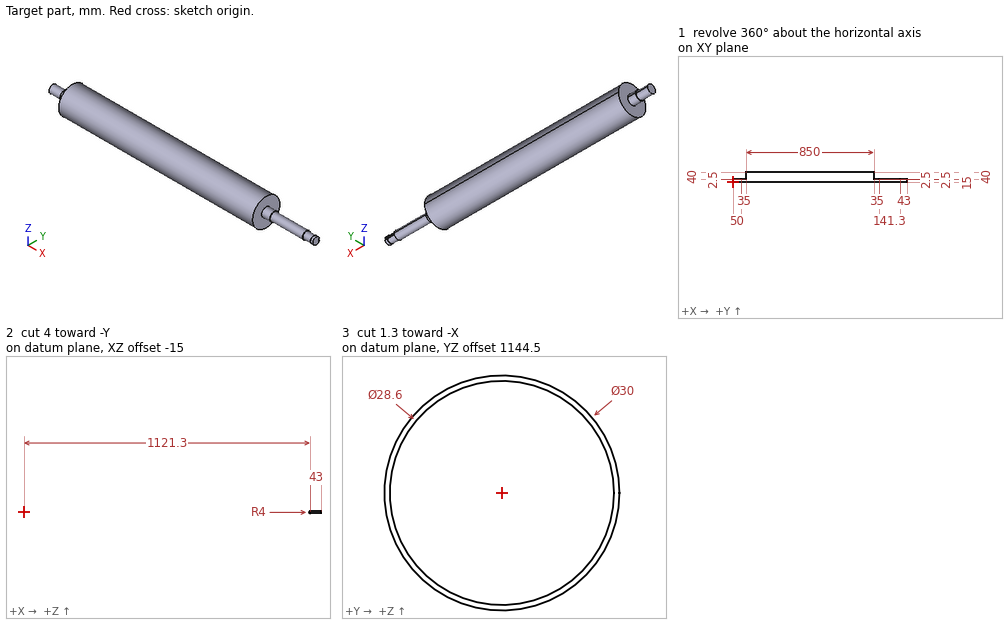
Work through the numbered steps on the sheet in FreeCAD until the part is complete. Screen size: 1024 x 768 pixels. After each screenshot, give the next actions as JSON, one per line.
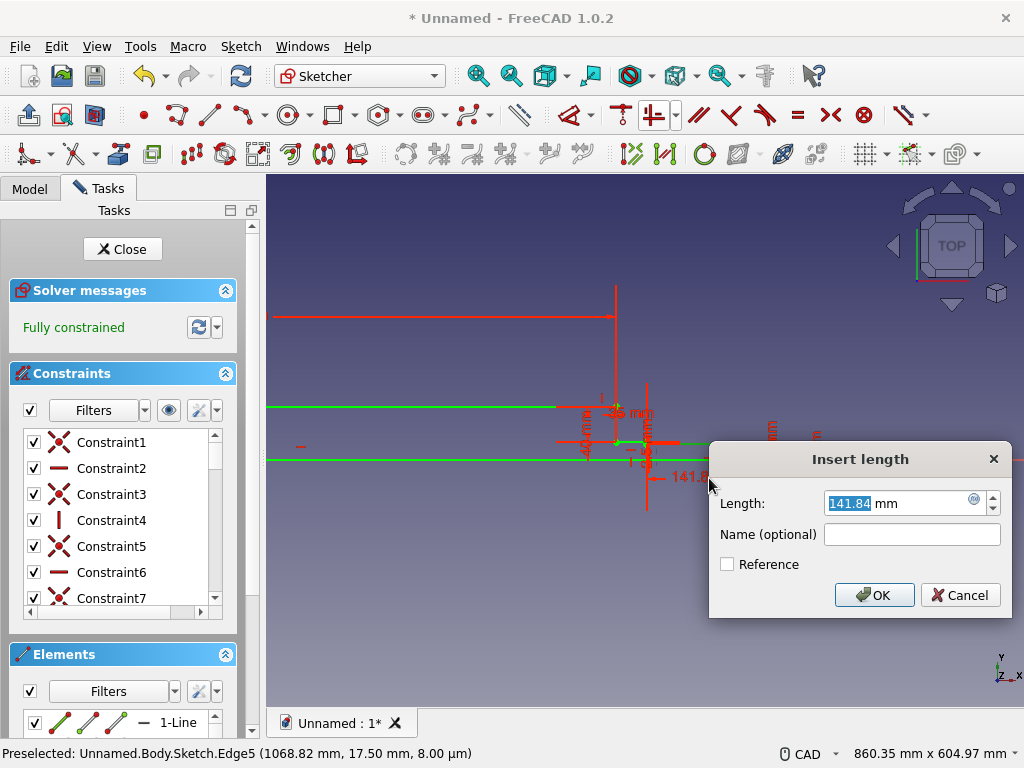
{"action": "type", "text": "141.3"}
{"action": "key", "text": "Return"}
{"action": "key", "text": "Escape"}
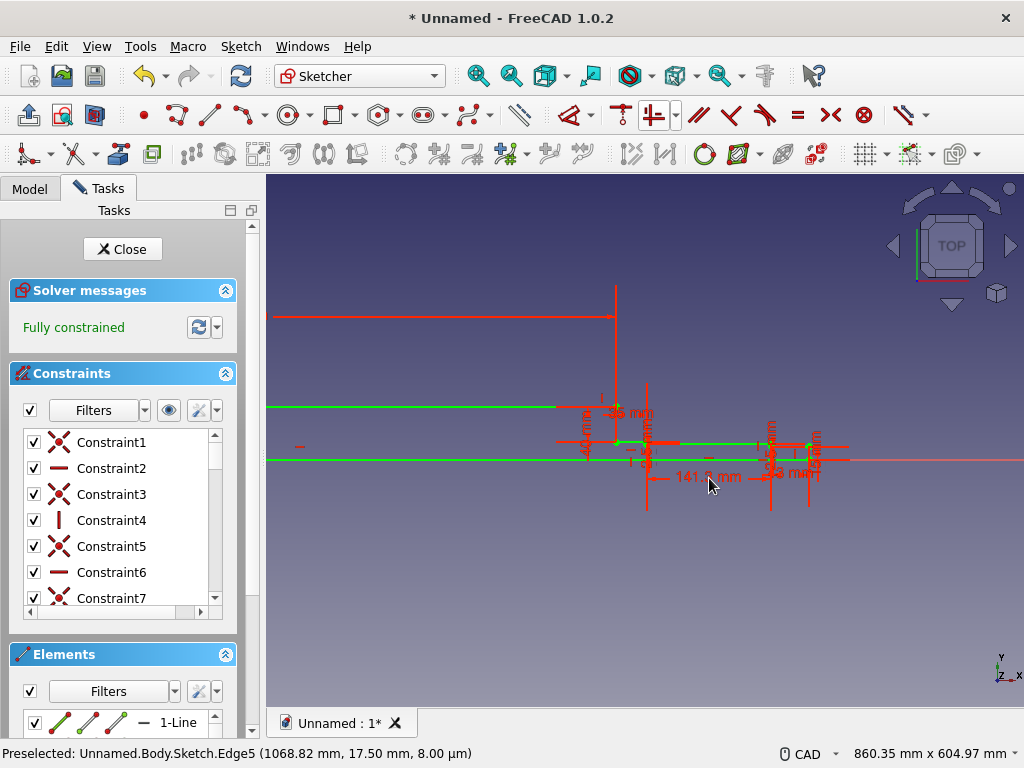
{"action": "left_click", "coordinate": [123, 249]}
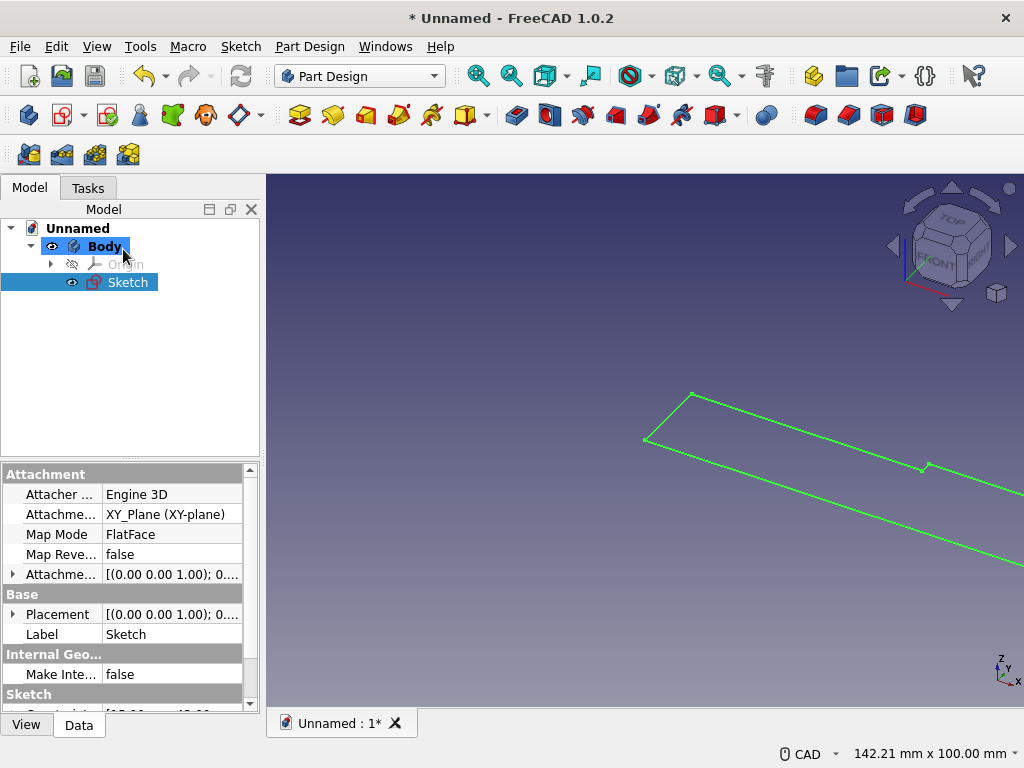
{"action": "left_click", "coordinate": [333, 116]}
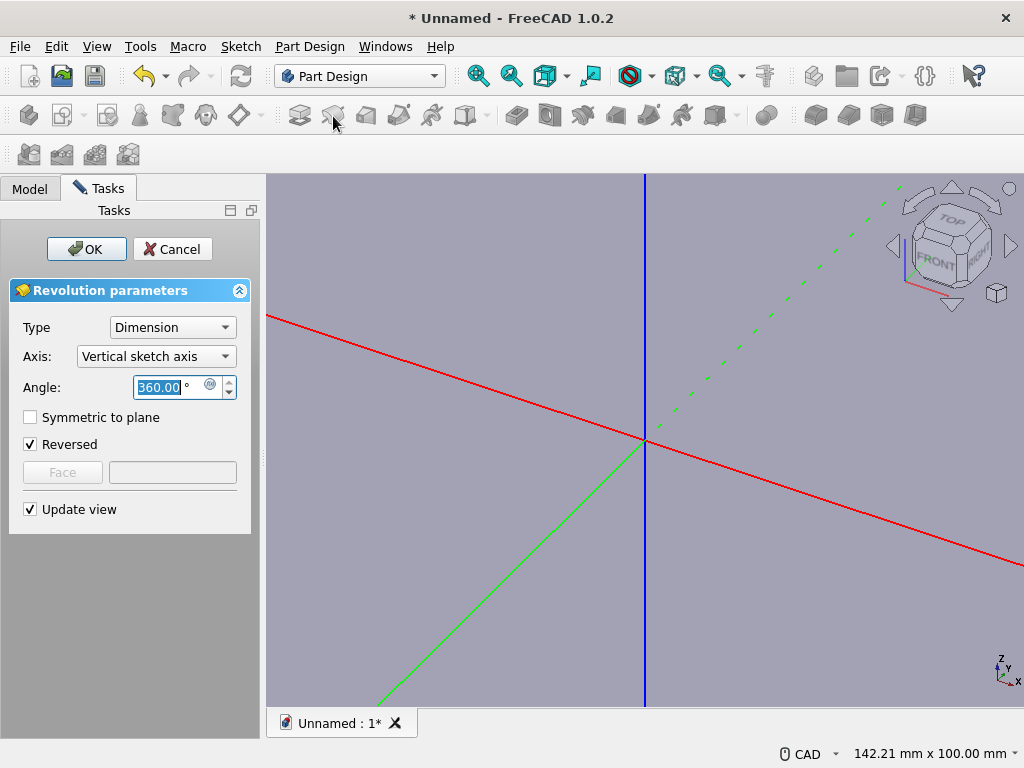
{"action": "left_click", "coordinate": [157, 356]}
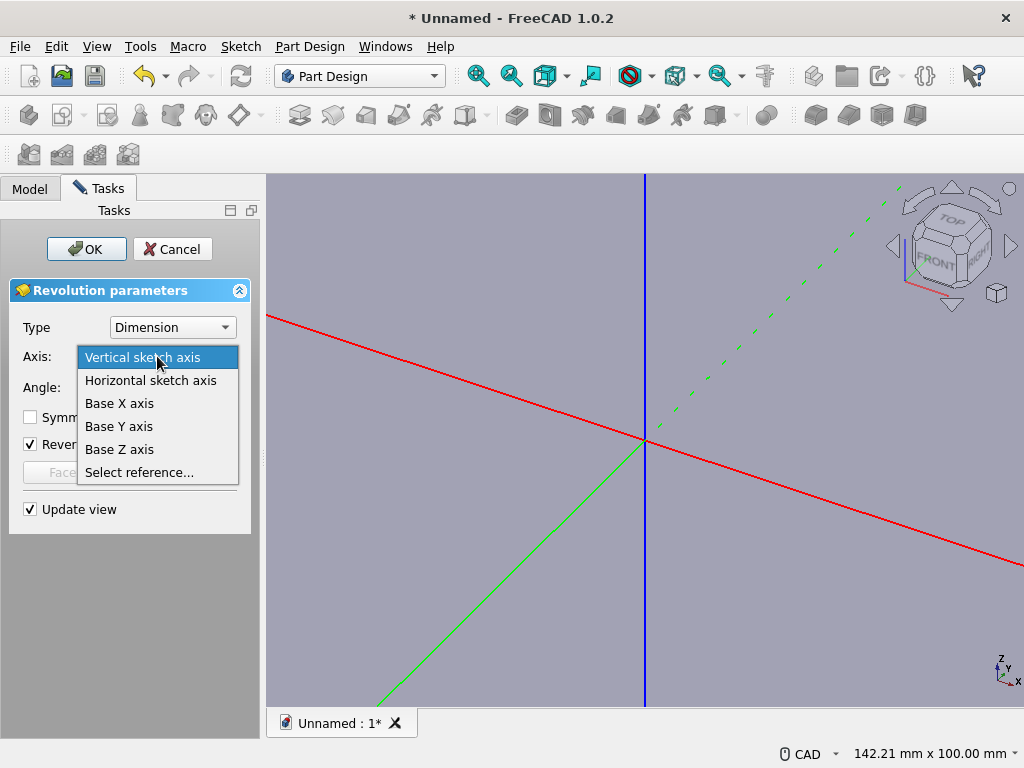
{"action": "left_click", "coordinate": [156, 380]}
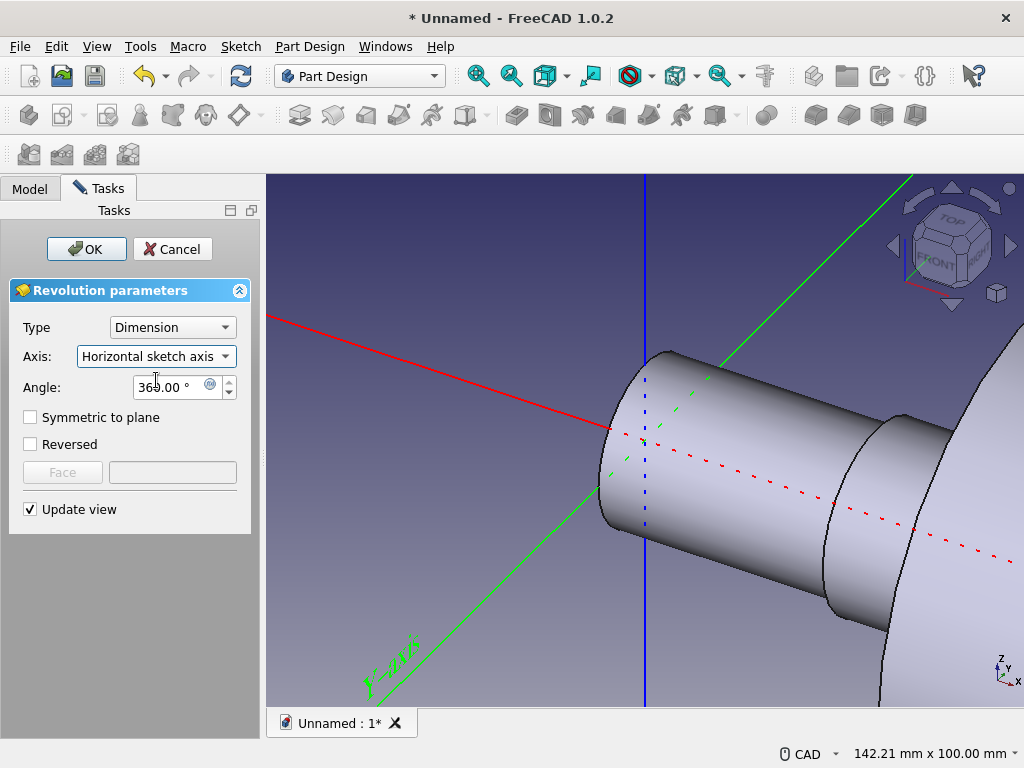
{"action": "left_click", "coordinate": [87, 249]}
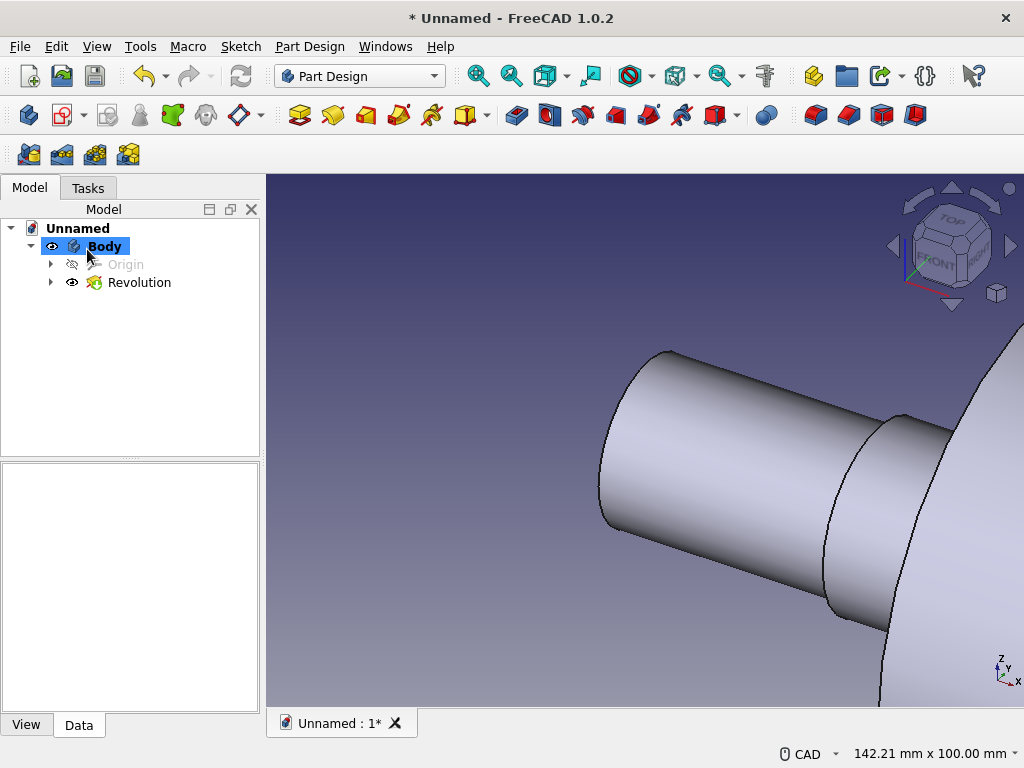
{"action": "key", "text": "v f"}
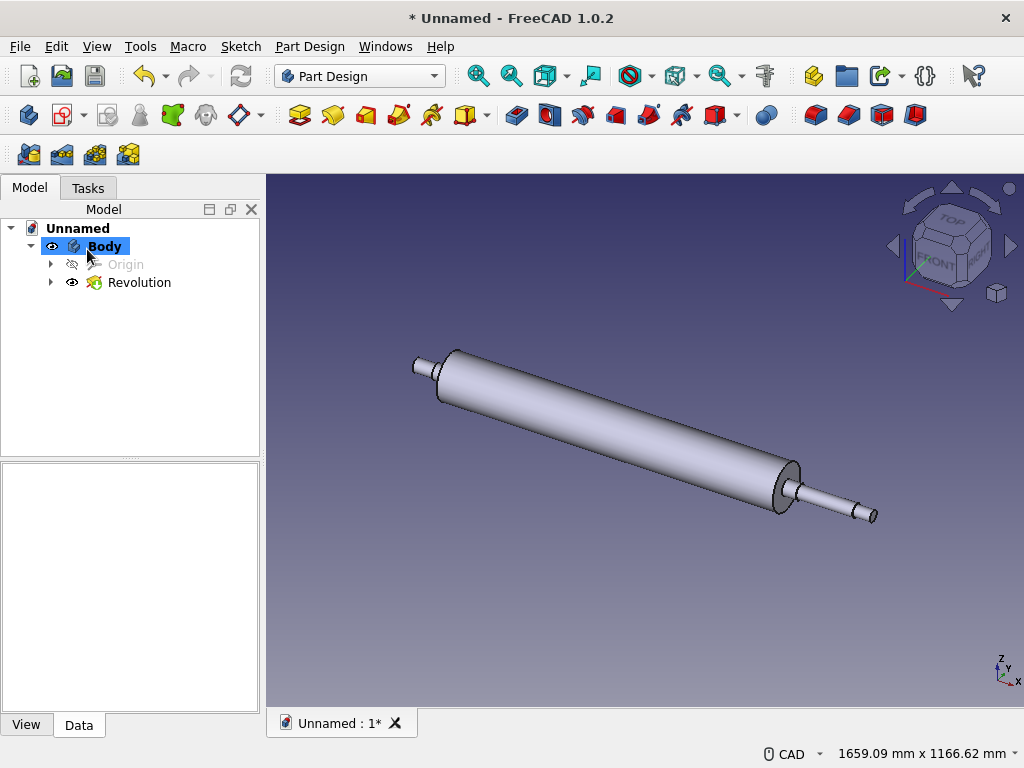
{"action": "left_click", "coordinate": [51, 264]}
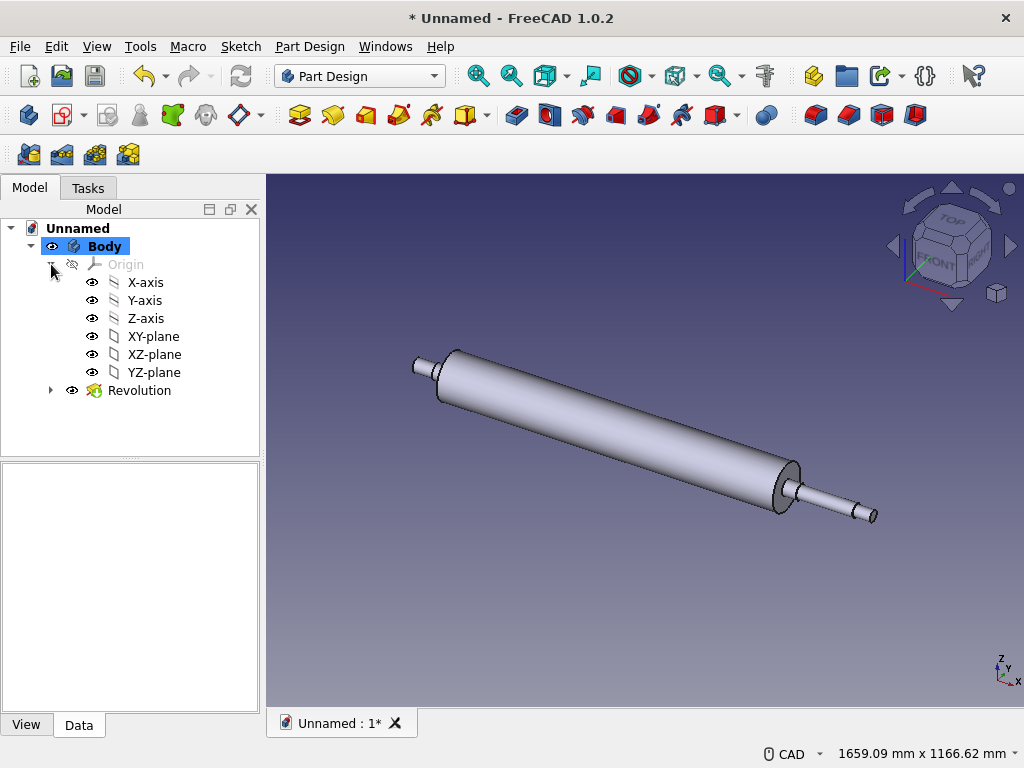
{"action": "left_click", "coordinate": [137, 354]}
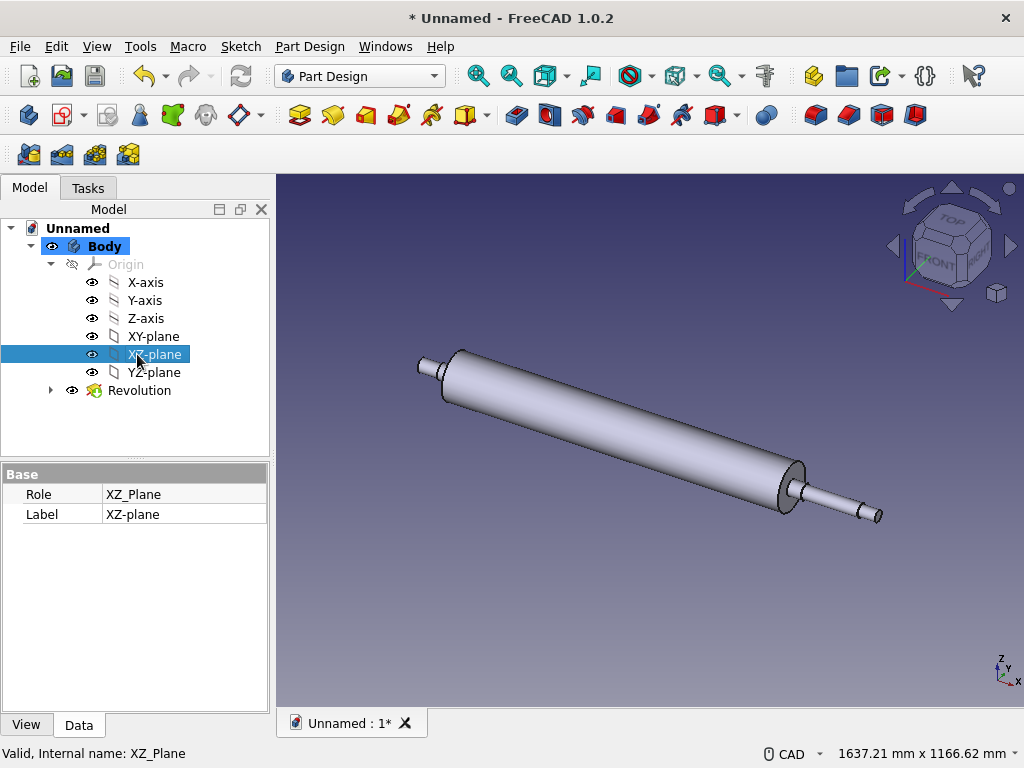
{"action": "left_click", "coordinate": [238, 116]}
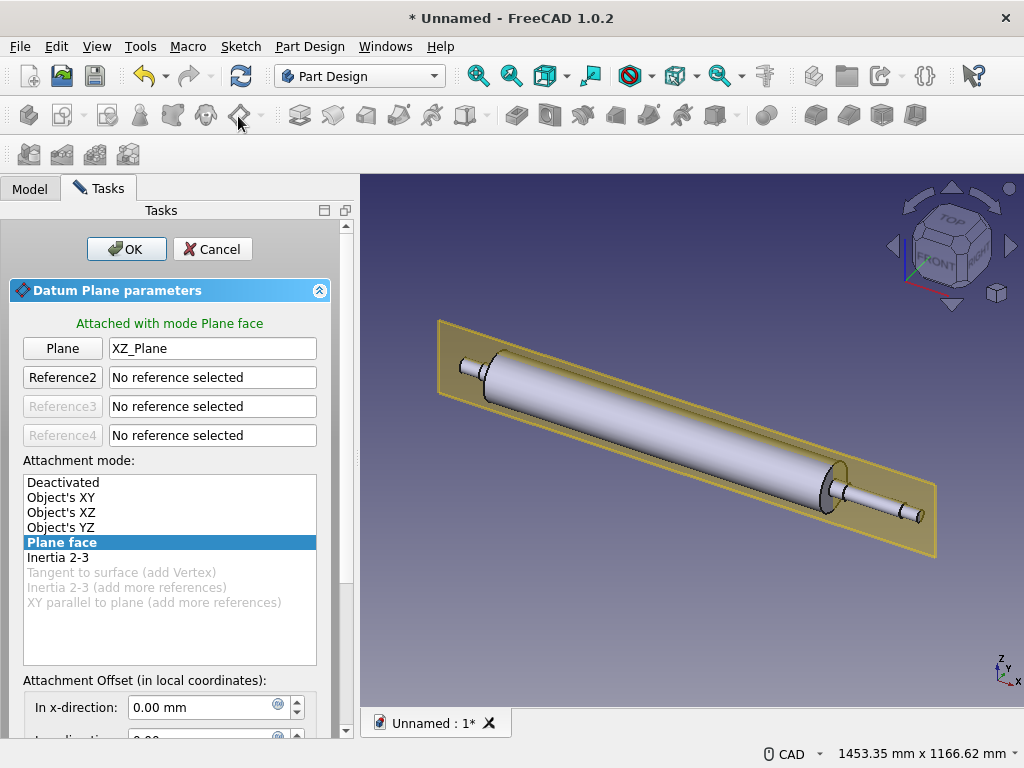
{"action": "scroll", "coordinate": [346, 479], "scroll_direction": "down", "scroll_amount": 2}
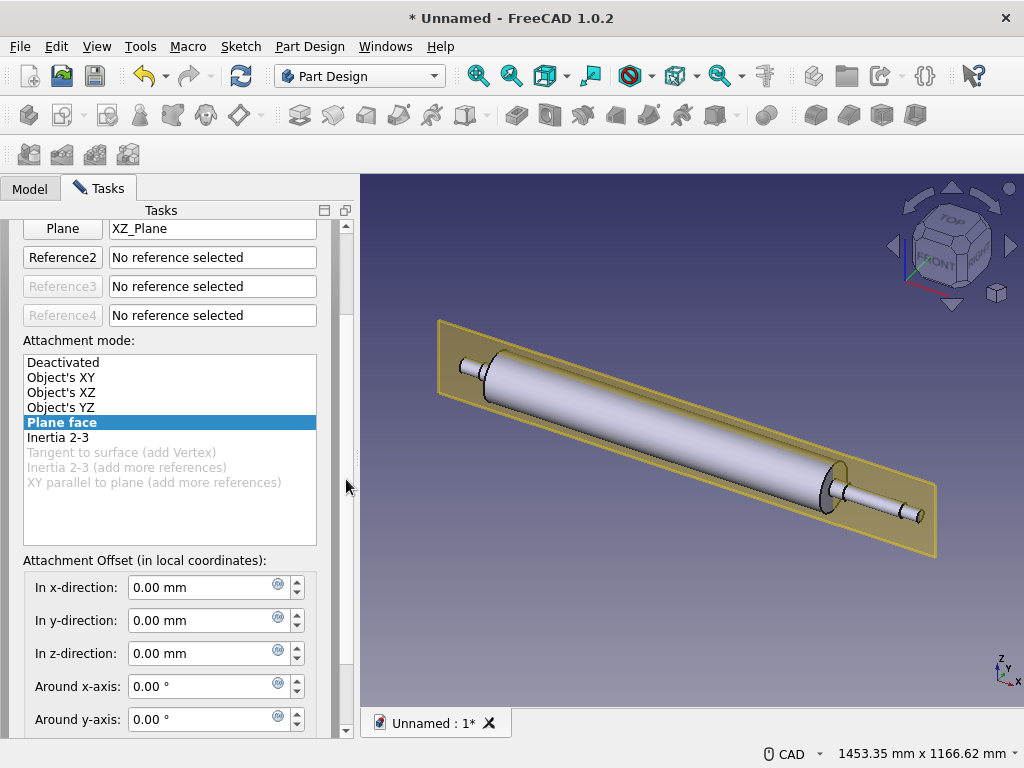
{"action": "triple_click", "coordinate": [210, 654]}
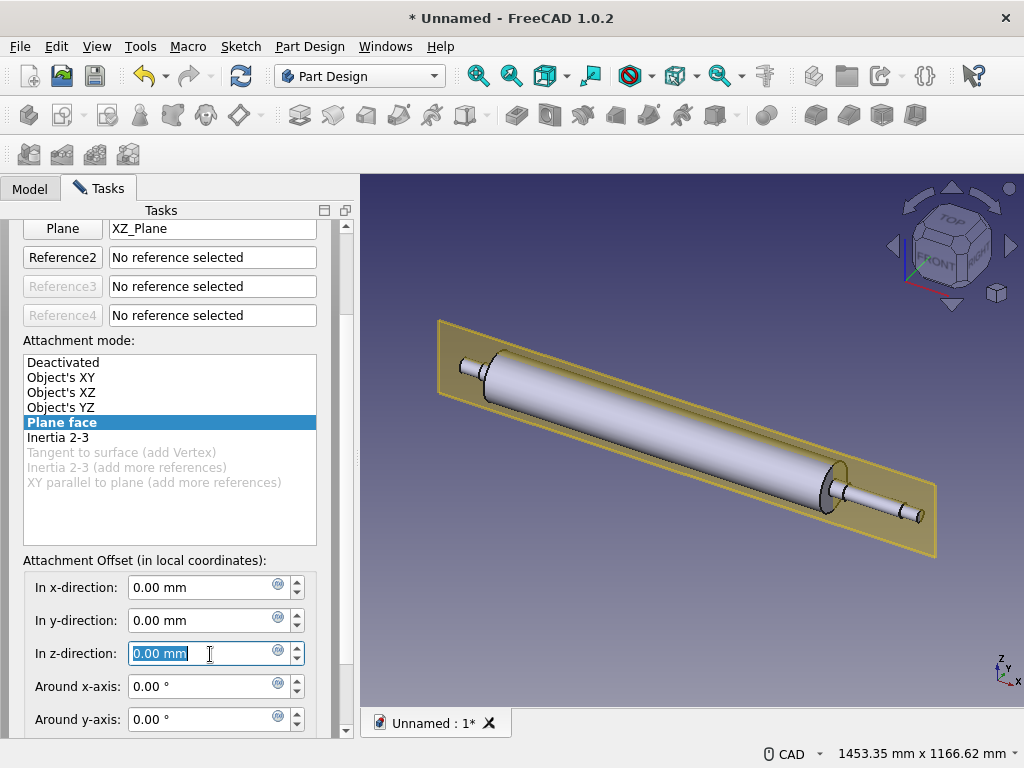
{"action": "type", "text": "-15"}
{"action": "key", "text": "Tab"}